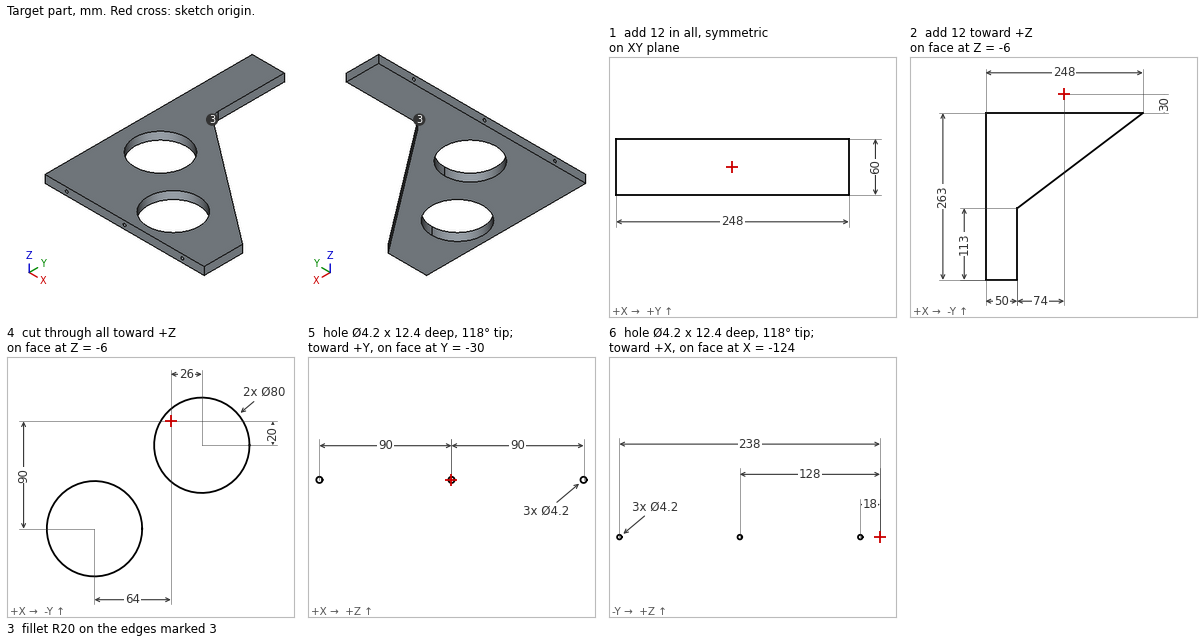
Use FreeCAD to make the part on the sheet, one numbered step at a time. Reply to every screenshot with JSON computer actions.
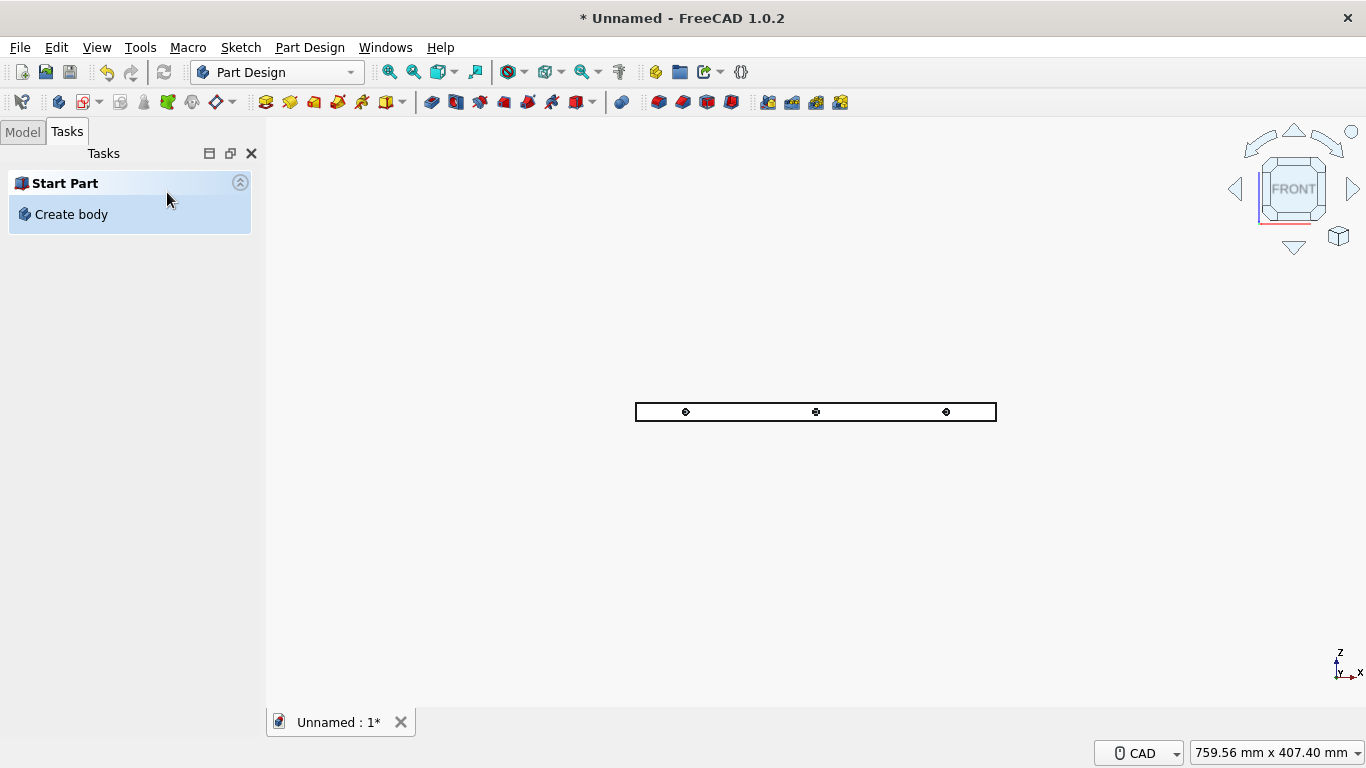
{"action": "key", "text": "v f"}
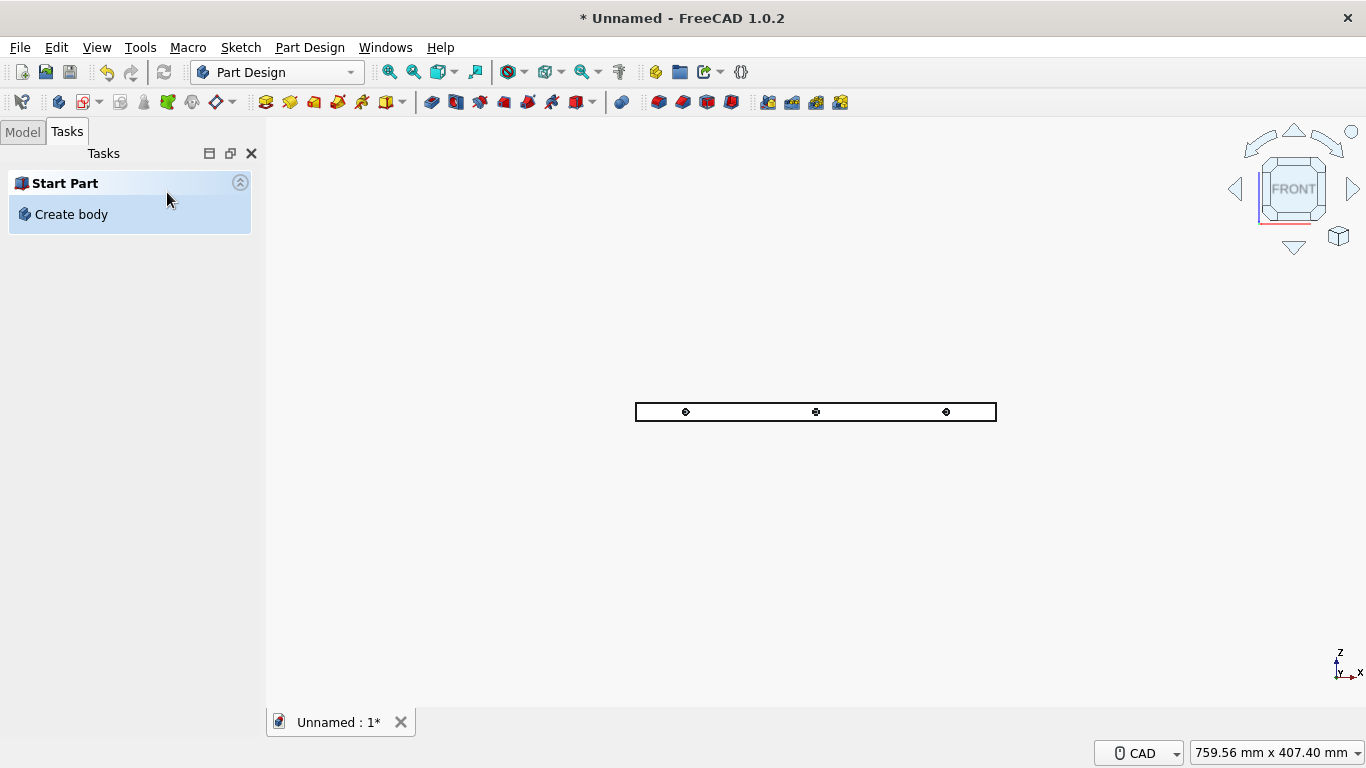
{"action": "key", "text": "6"}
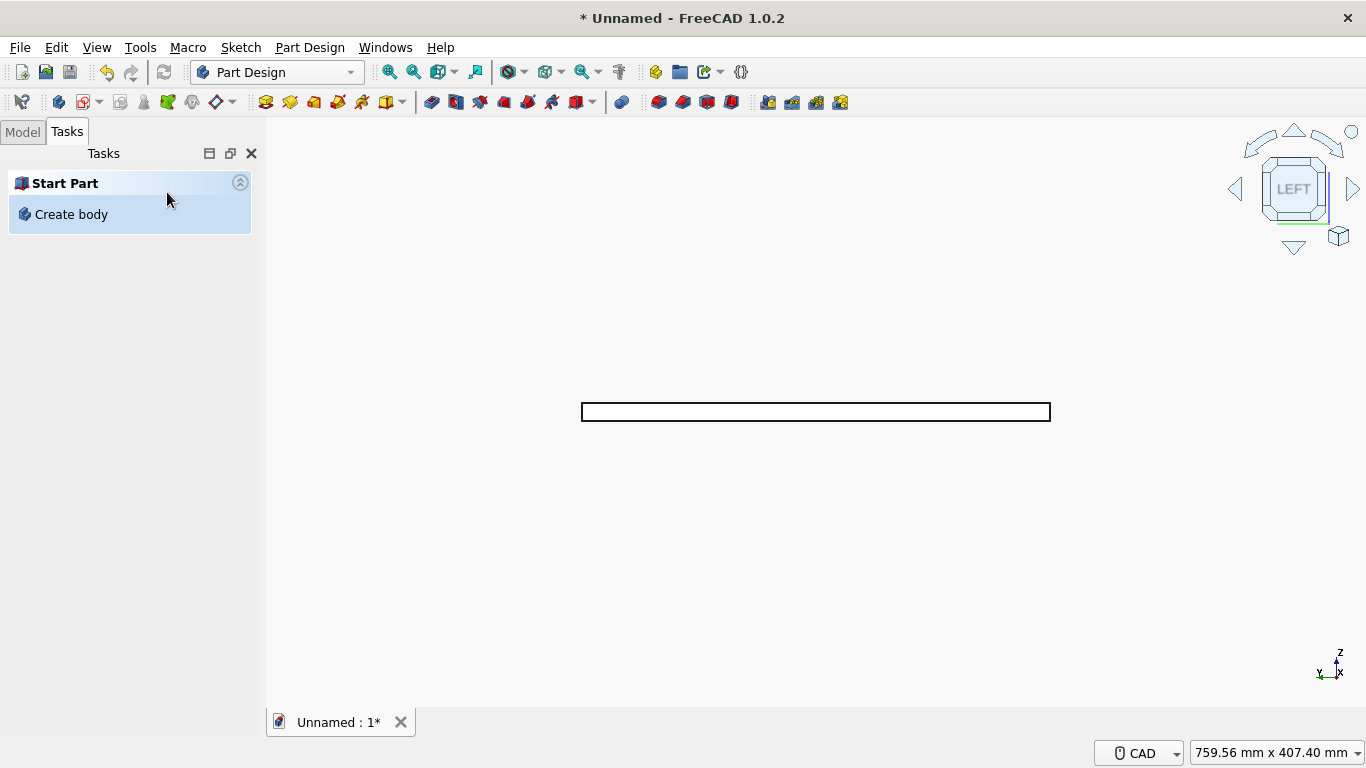
{"action": "key", "text": "v f"}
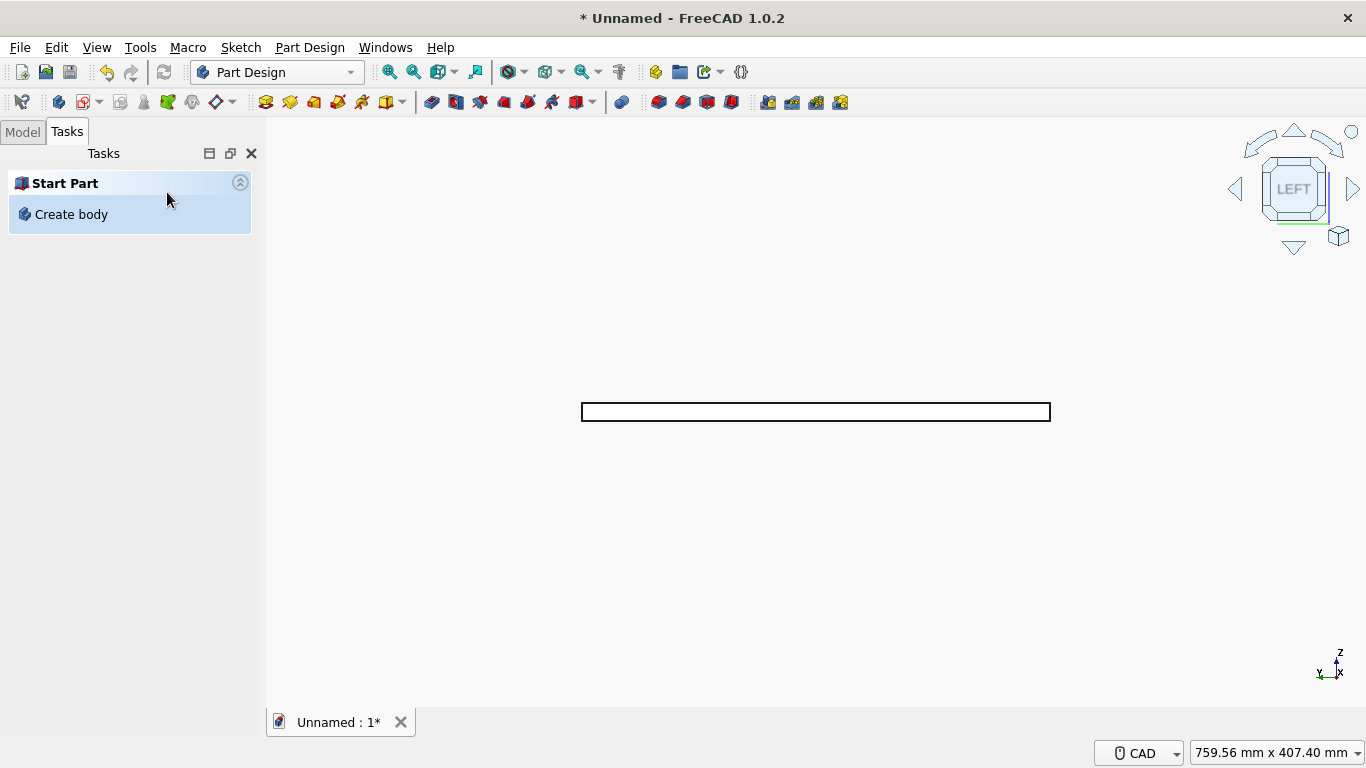
{"action": "left_click", "coordinate": [616, 411]}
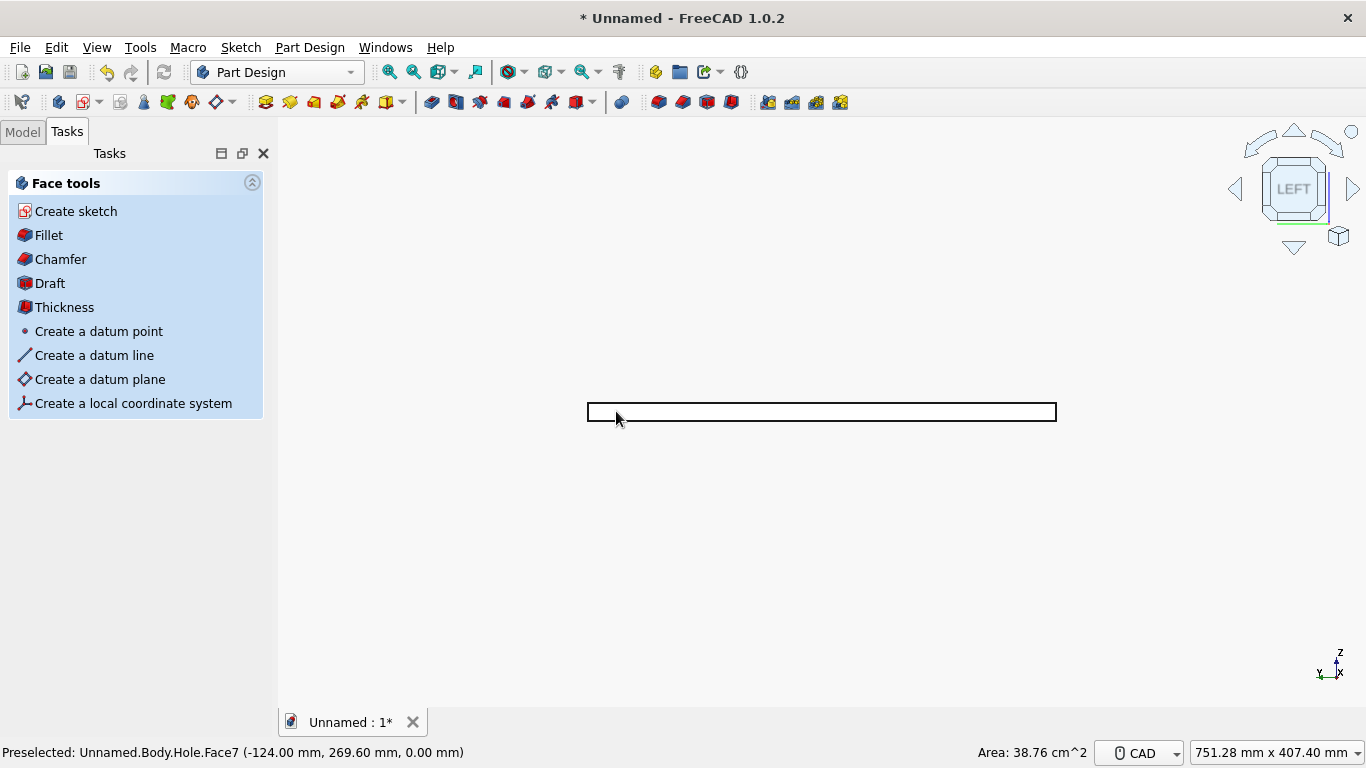
{"action": "left_click", "coordinate": [84, 102]}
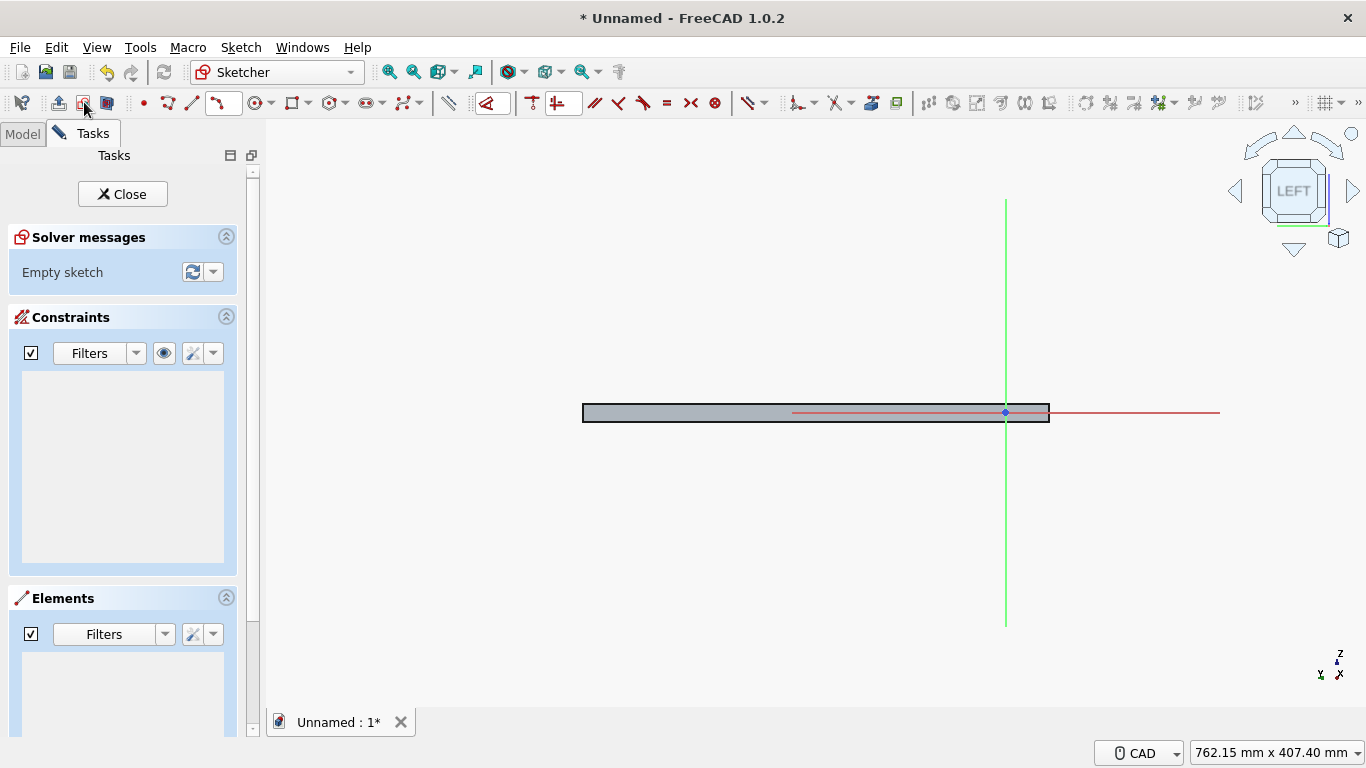
{"action": "scroll", "coordinate": [936, 413], "scroll_direction": "up", "scroll_amount": 3}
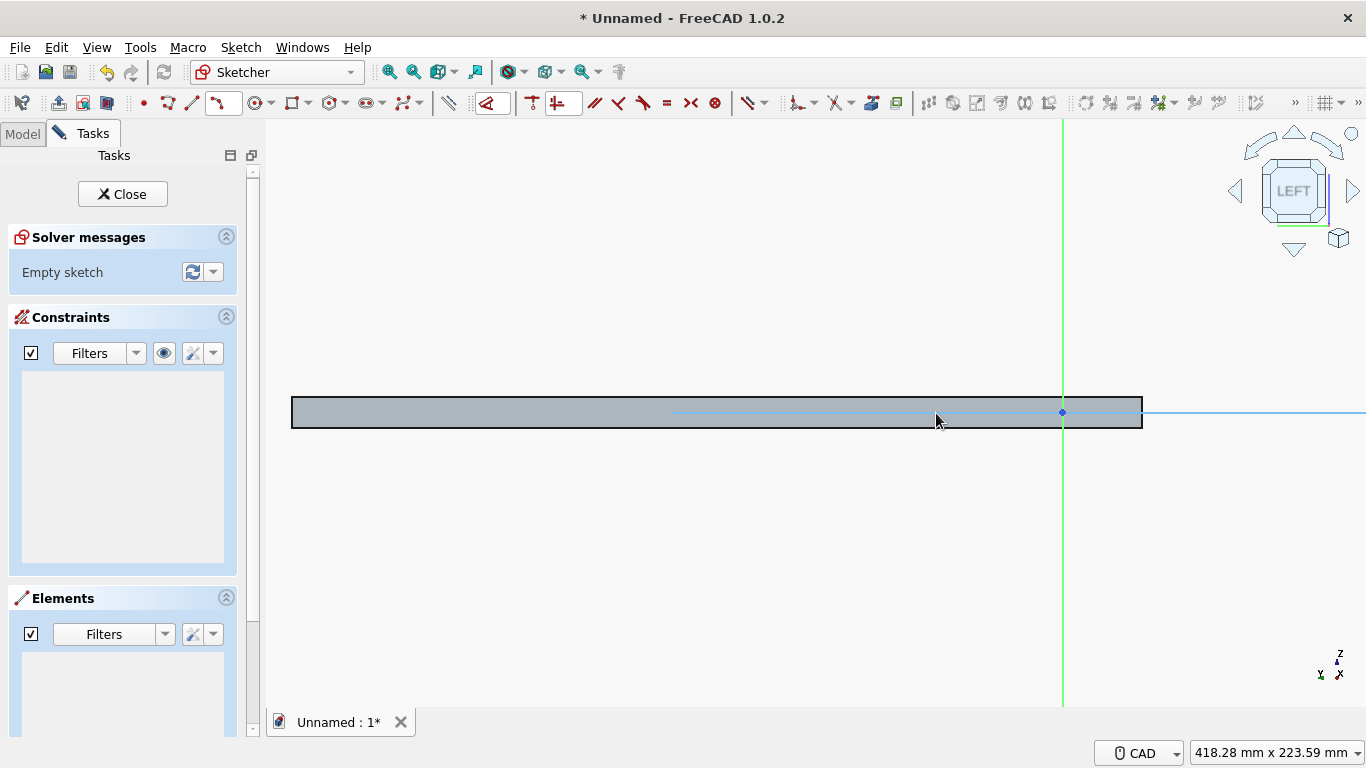
{"action": "key", "text": "g c"}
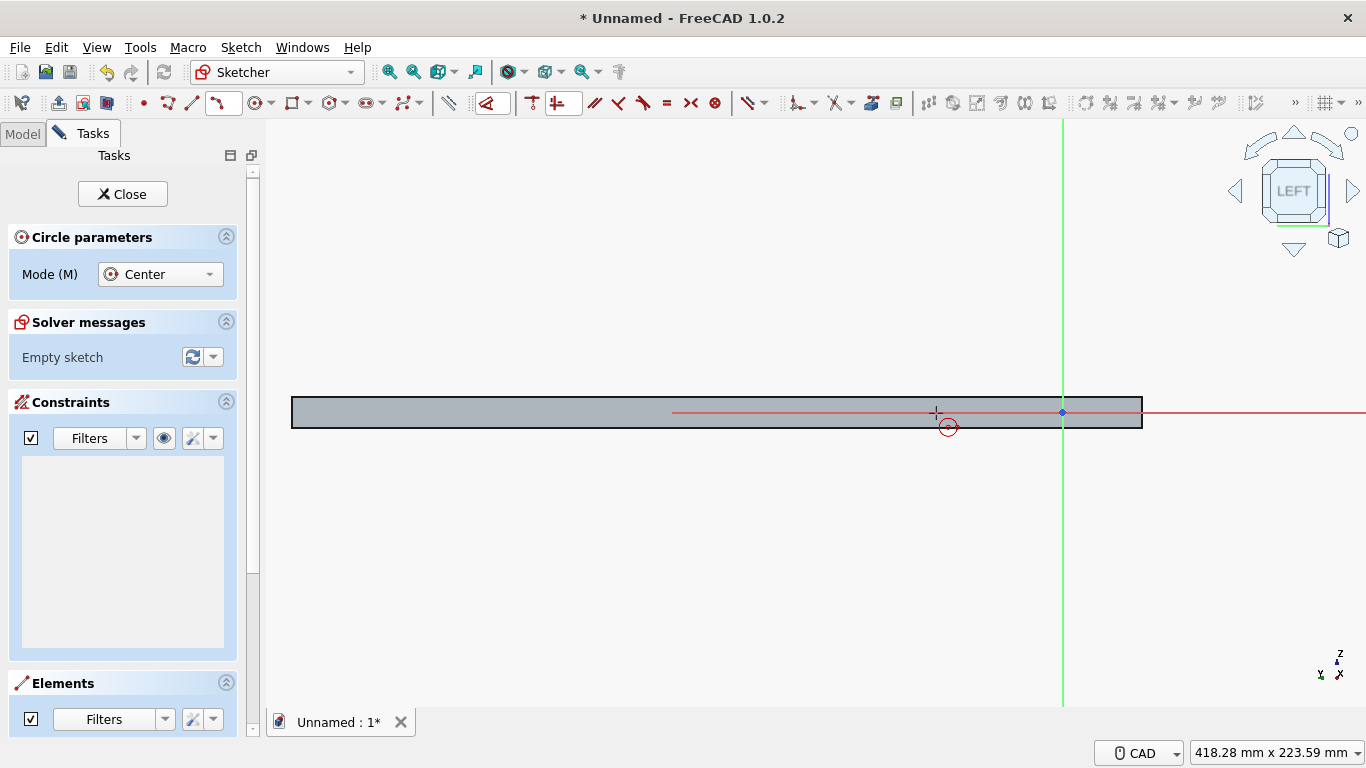
{"action": "scroll", "coordinate": [437, 413], "scroll_direction": "up", "scroll_amount": 8}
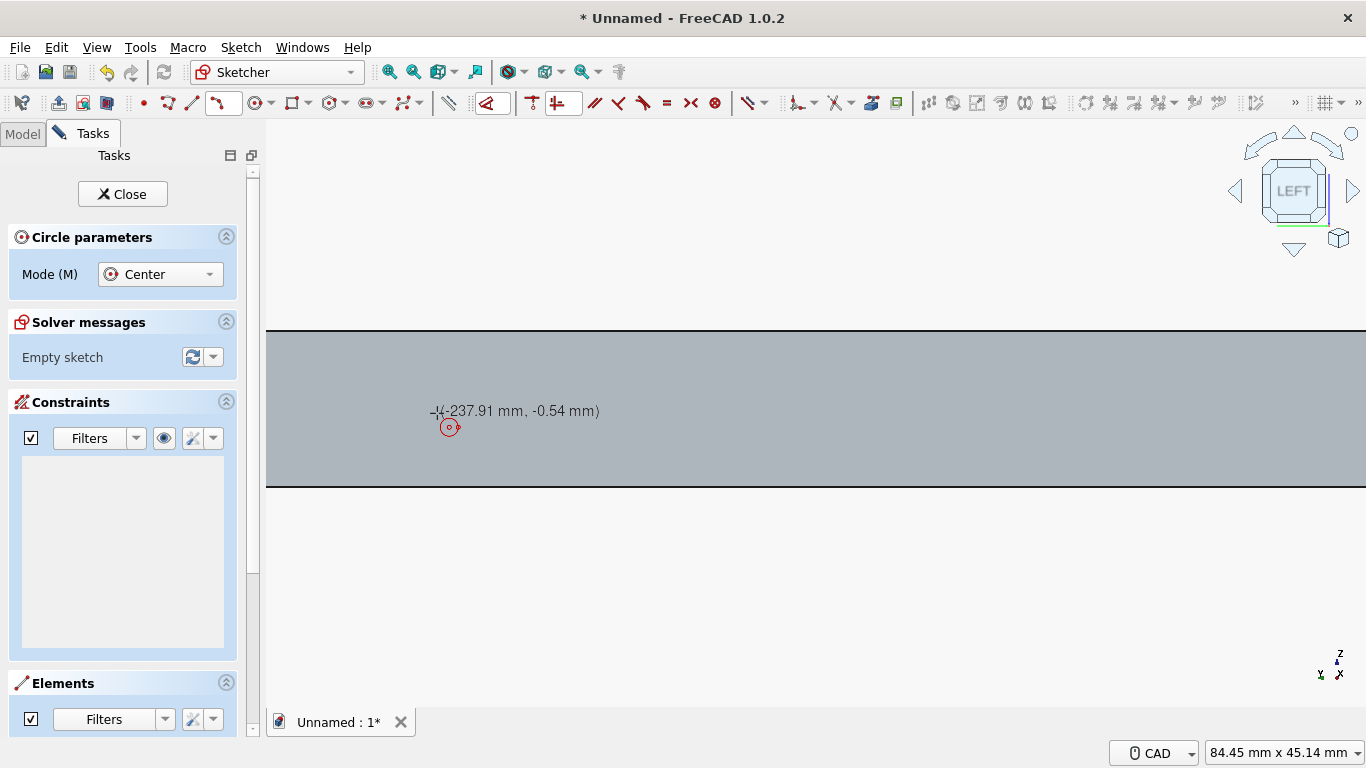
{"action": "scroll", "coordinate": [438, 414], "scroll_direction": "down", "scroll_amount": 8}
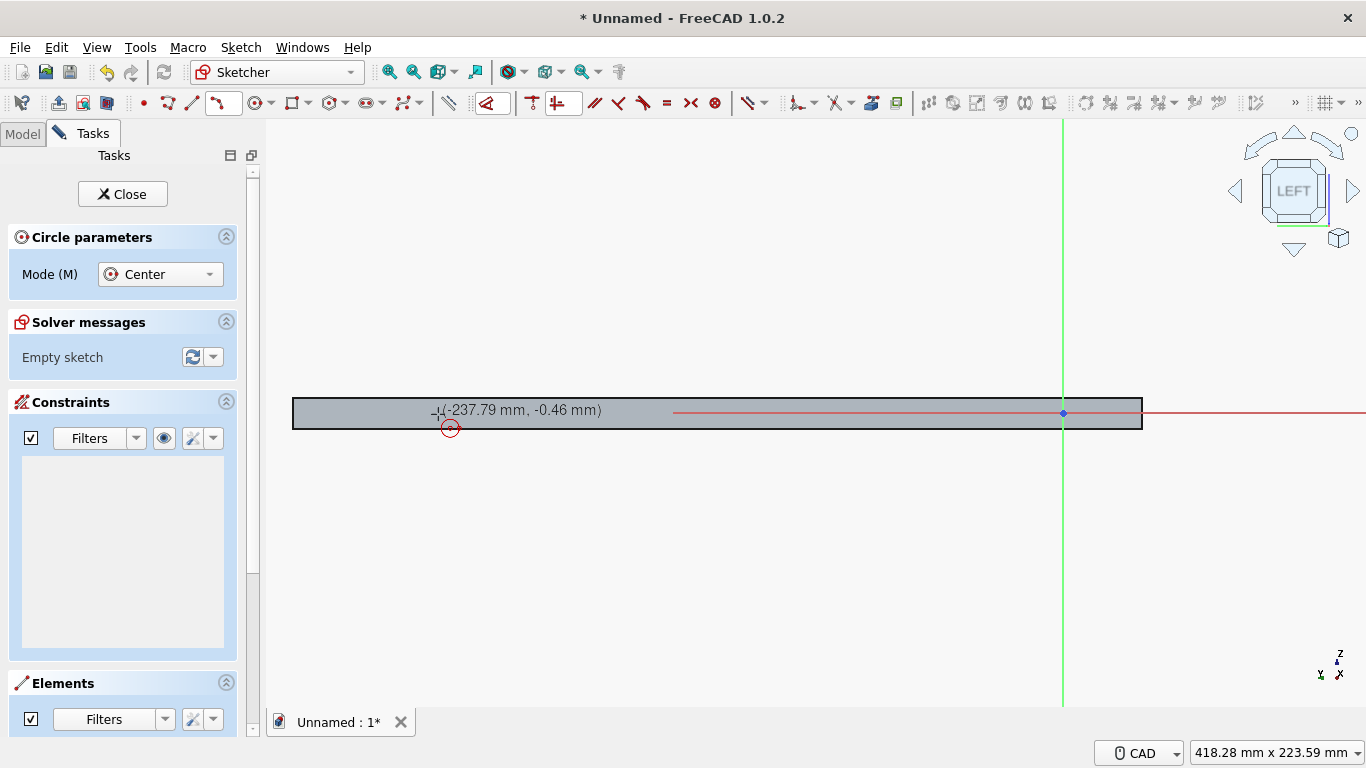
{"action": "left_click", "coordinate": [438, 413]}